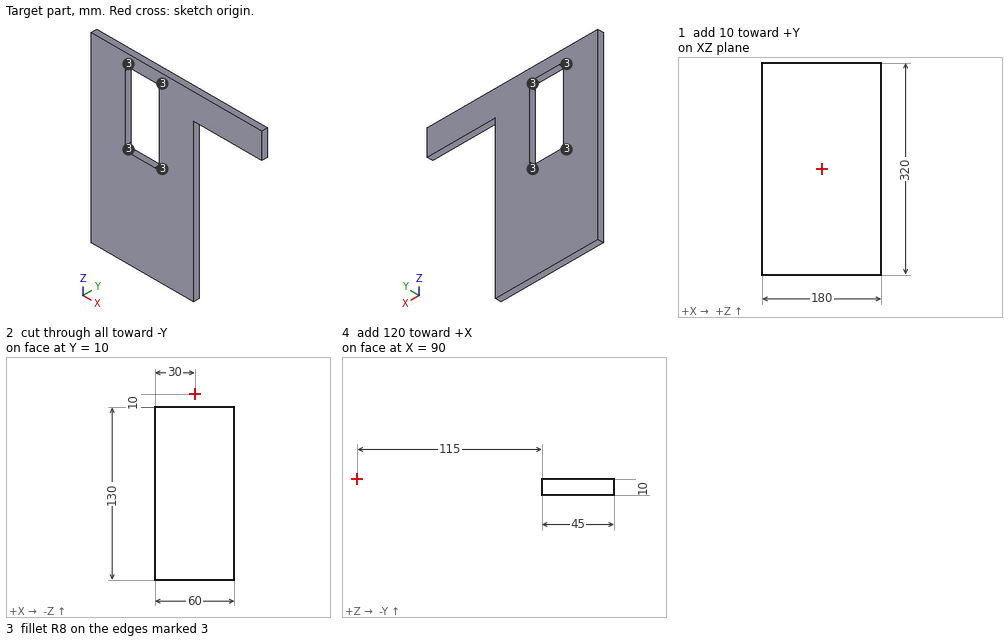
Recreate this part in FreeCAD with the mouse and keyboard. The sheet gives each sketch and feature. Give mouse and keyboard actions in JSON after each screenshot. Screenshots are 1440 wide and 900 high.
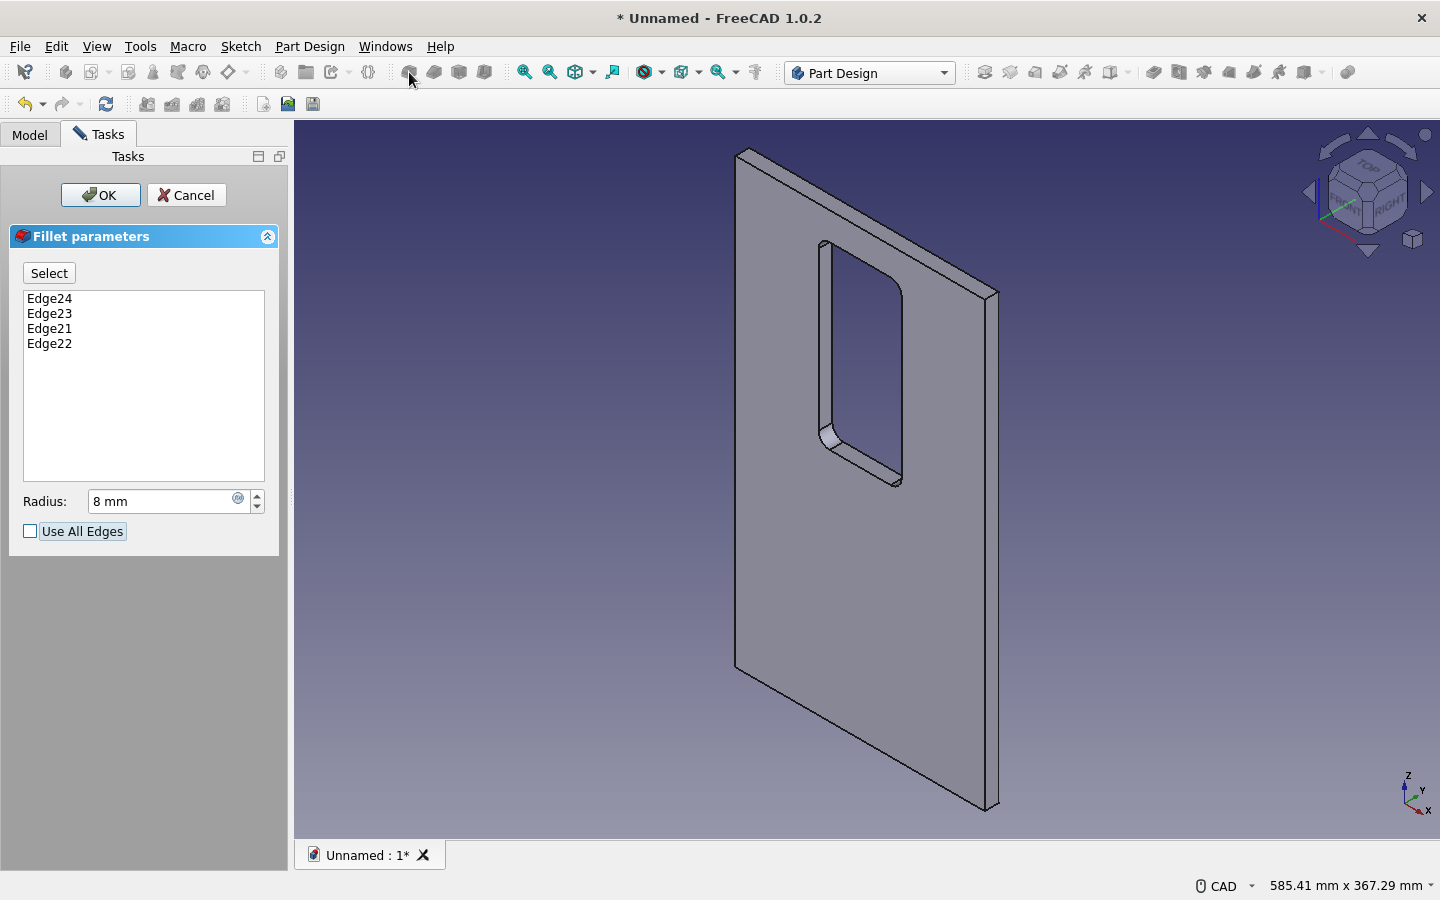
{"action": "left_click", "coordinate": [101, 195]}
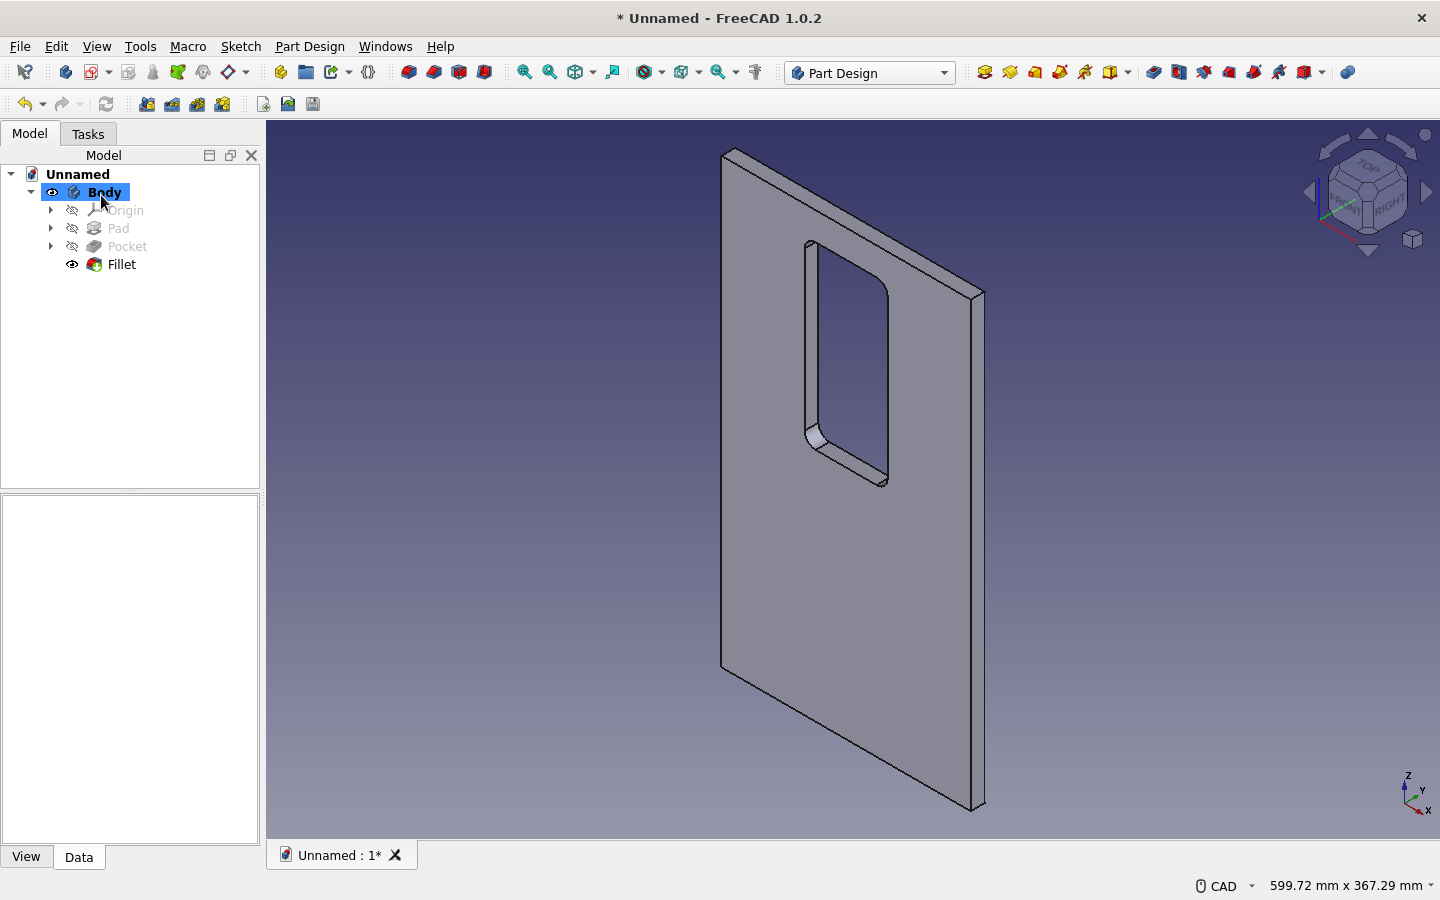
{"action": "key", "text": "3"}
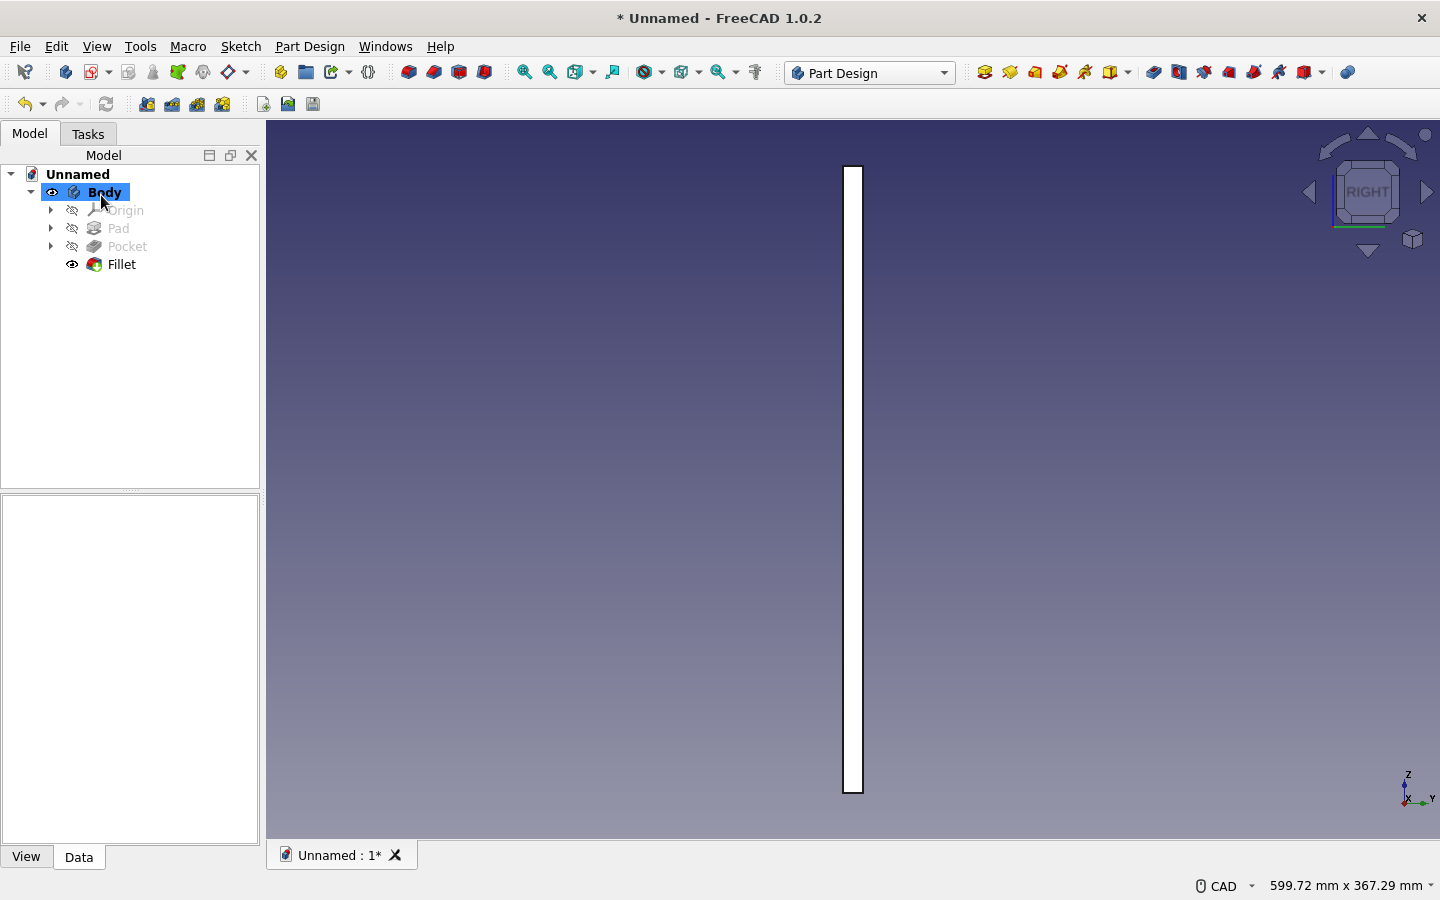
{"action": "left_click", "coordinate": [853, 478]}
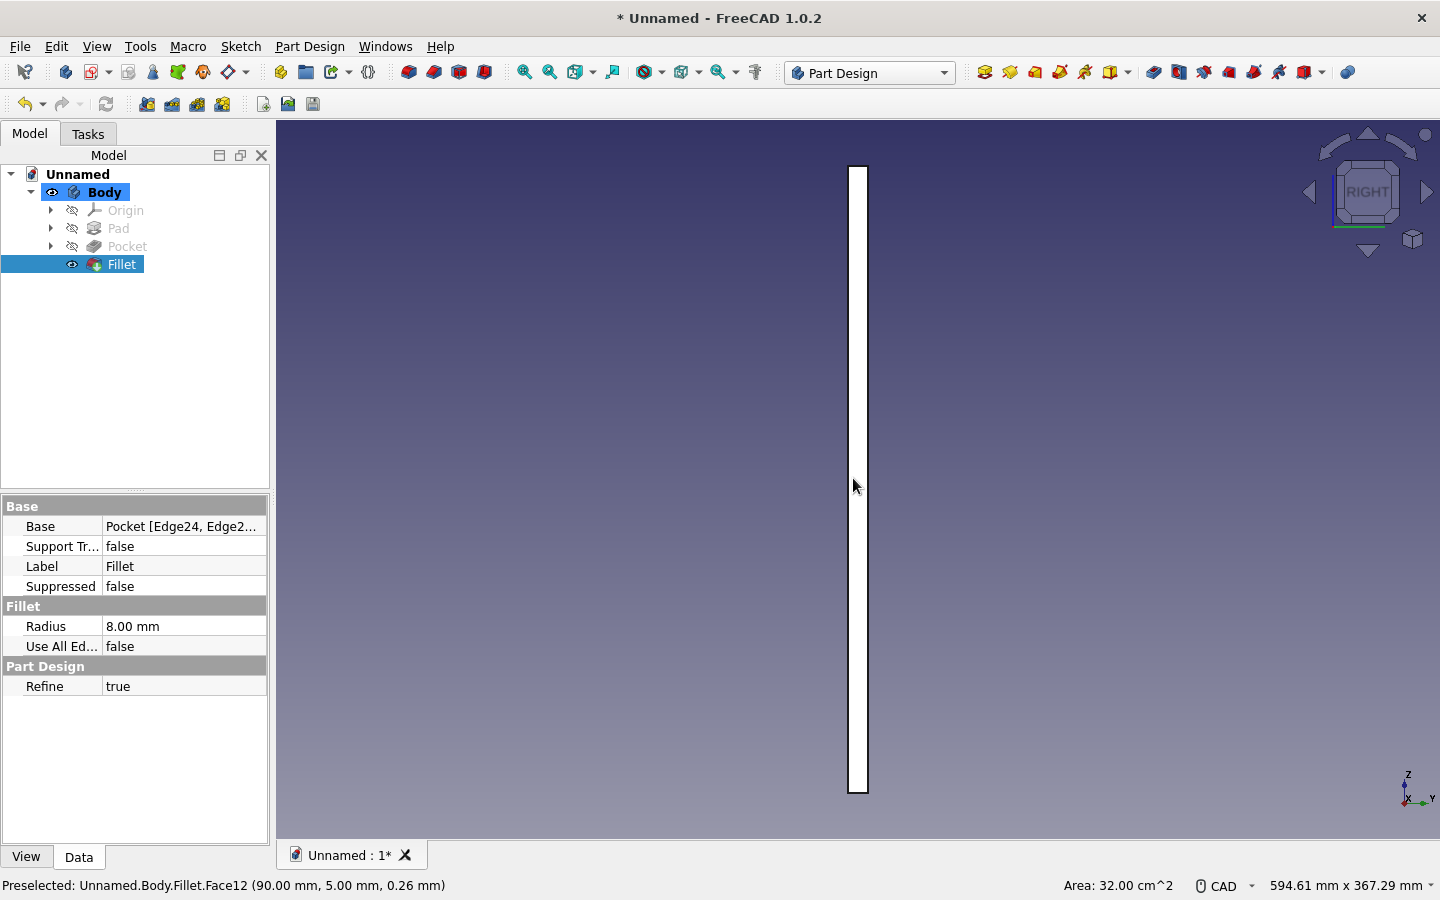
{"action": "left_click", "coordinate": [90, 72]}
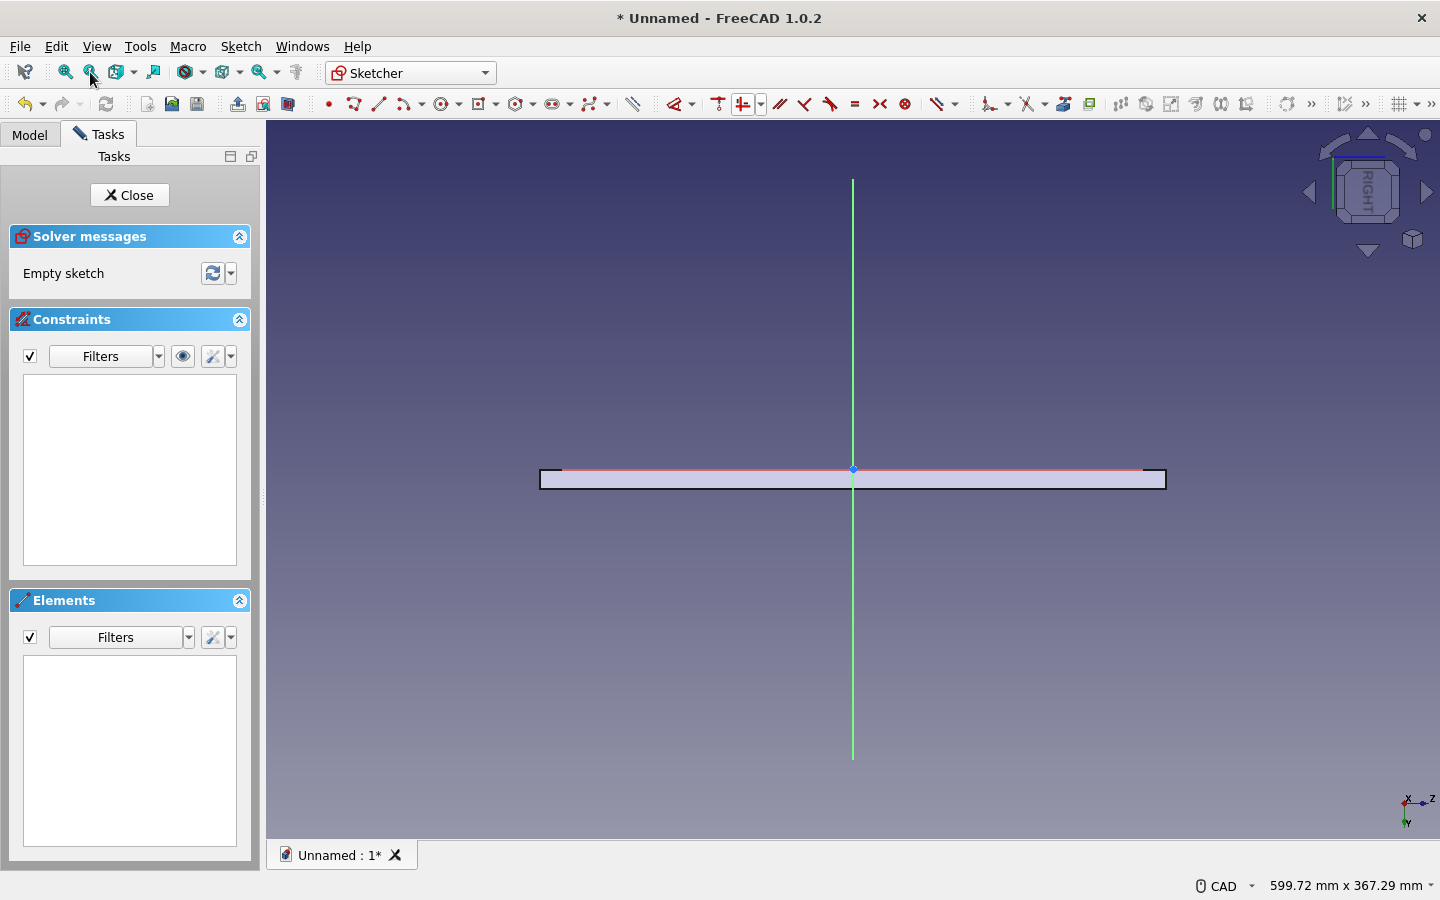
{"action": "scroll", "coordinate": [1175, 479], "scroll_direction": "up", "scroll_amount": 10}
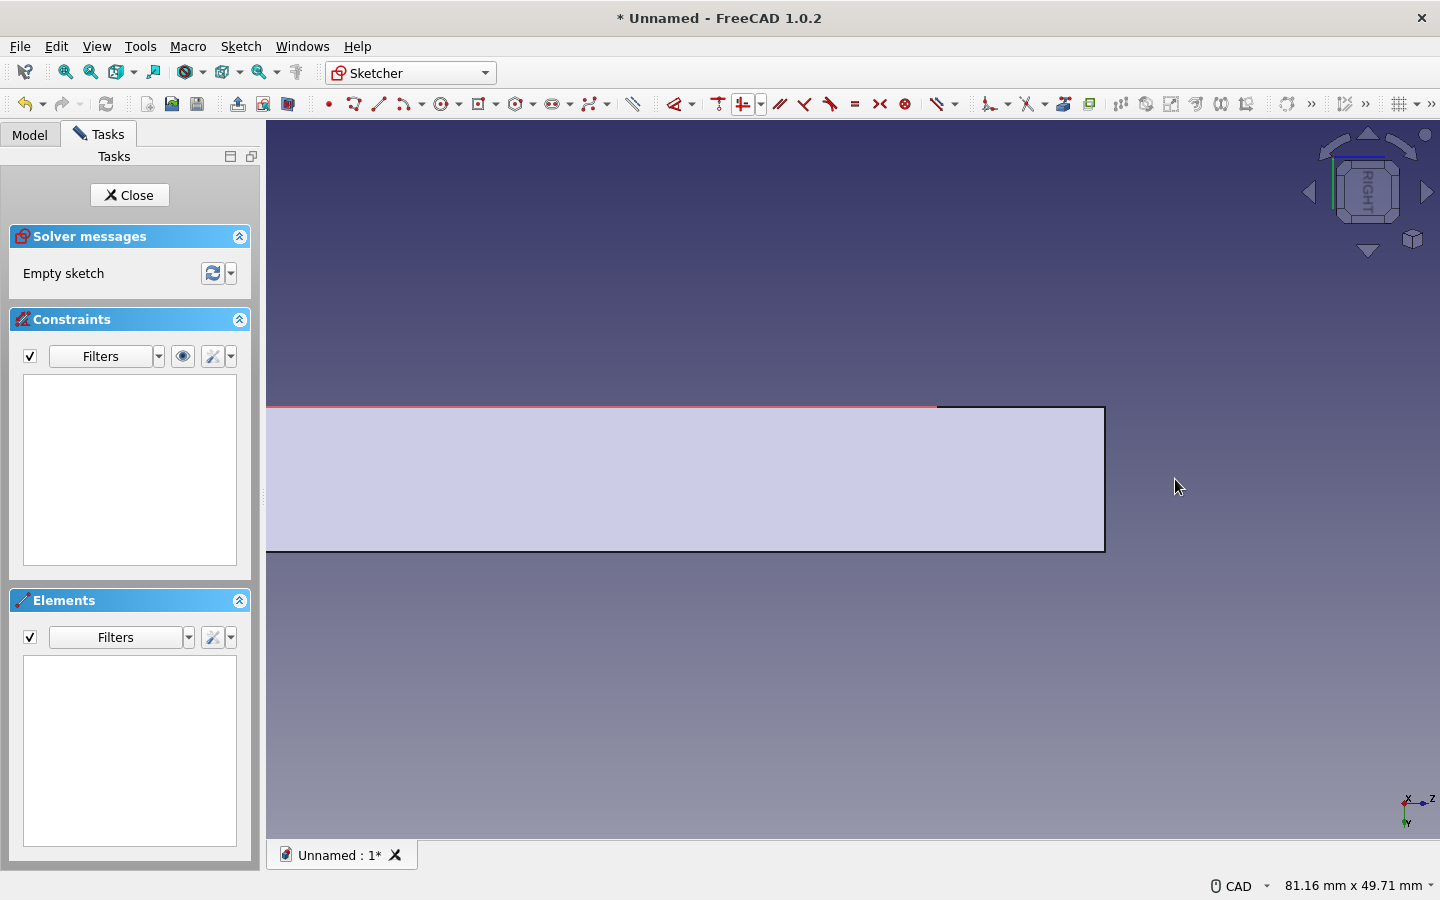
{"action": "key", "text": "g r"}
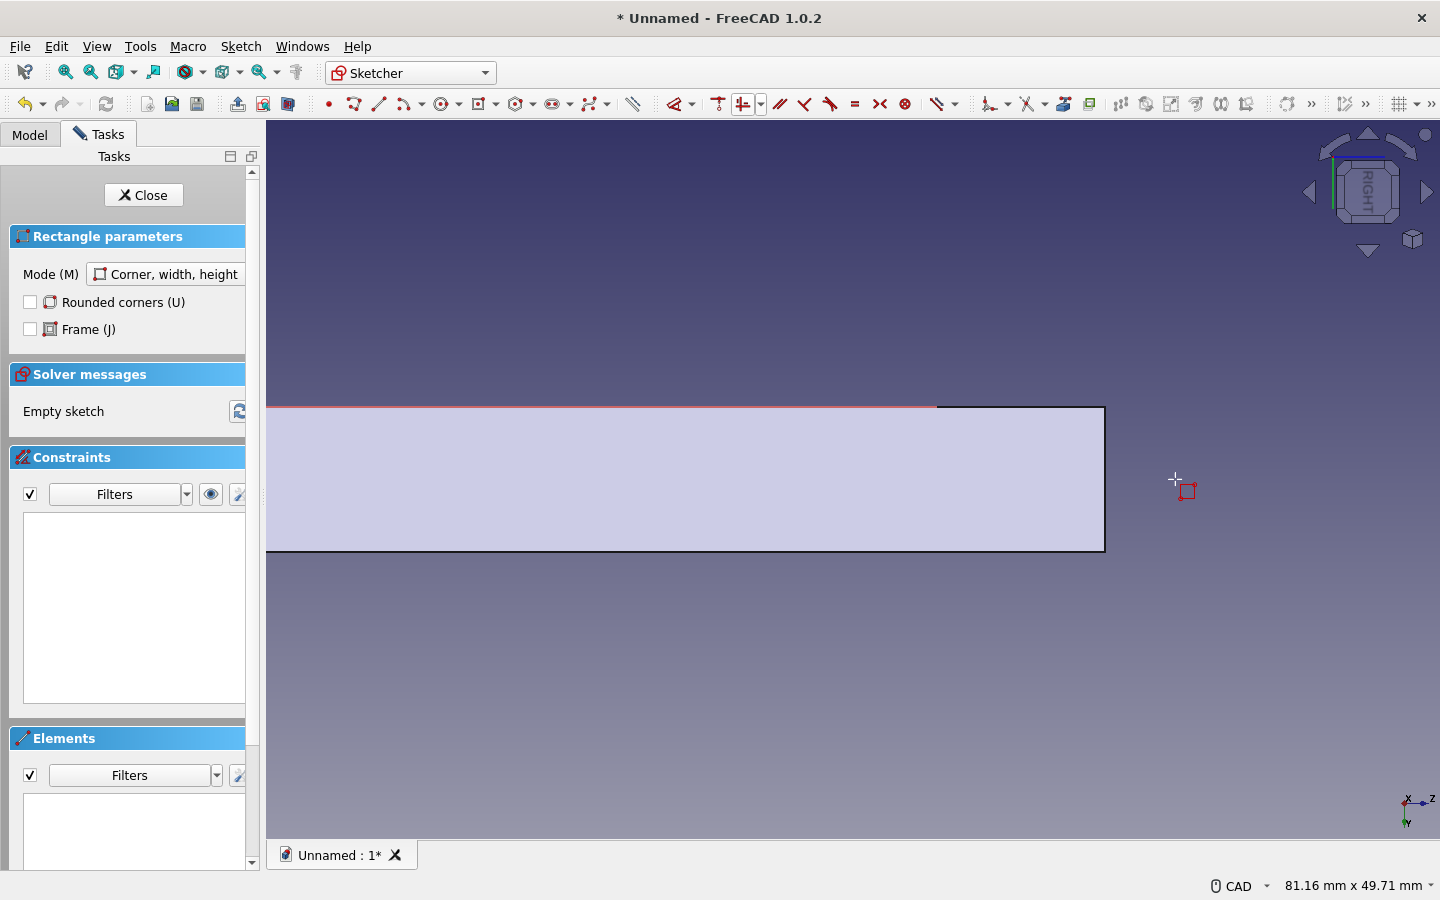
{"action": "left_click", "coordinate": [454, 407]}
{"action": "left_click", "coordinate": [1105, 552]}
{"action": "key", "text": "Escape"}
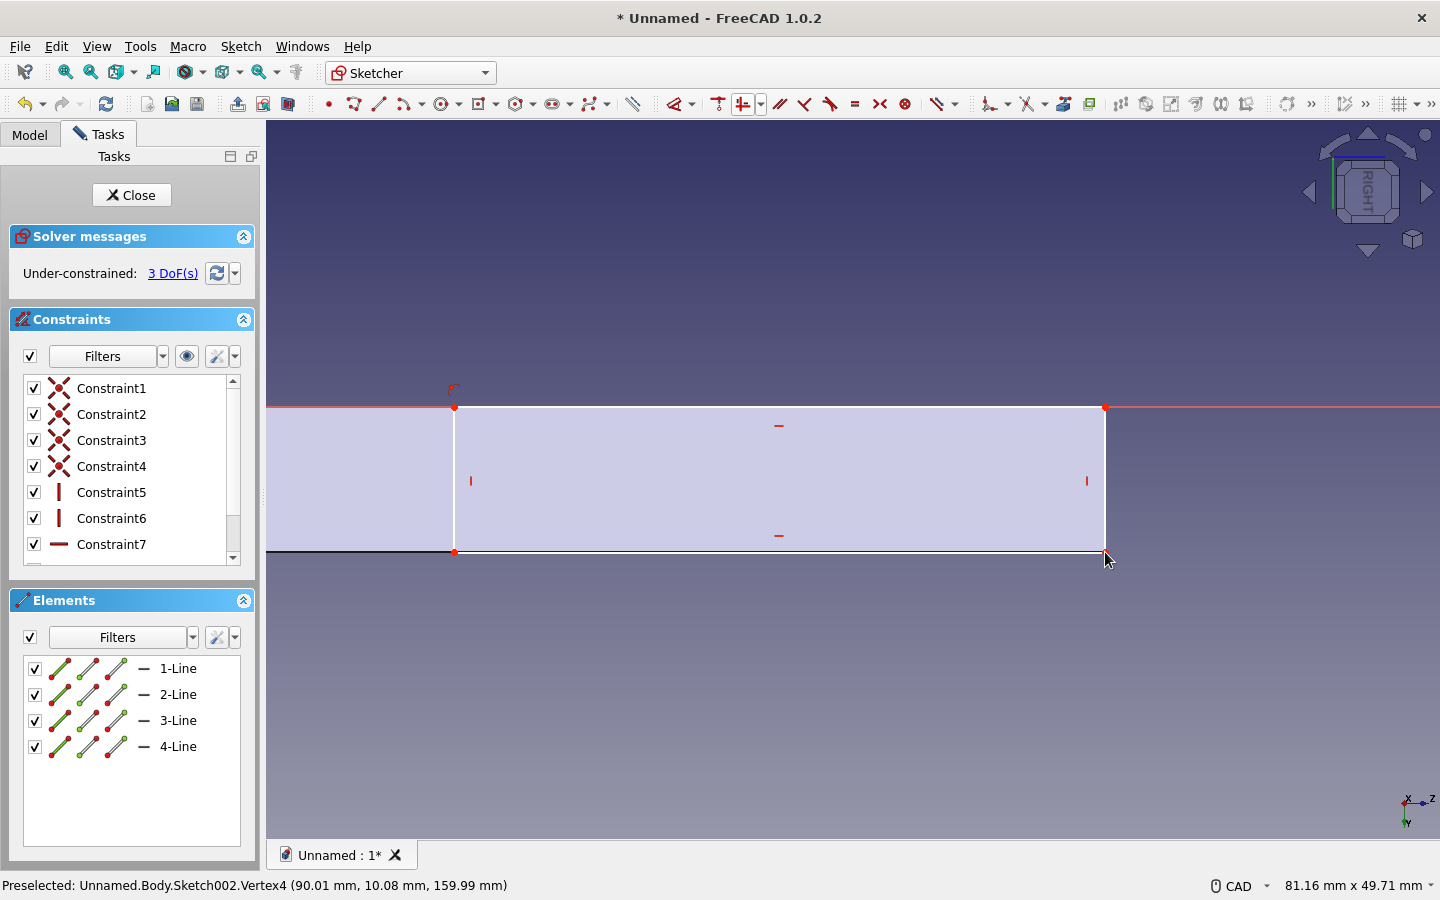
{"action": "key", "text": "d"}